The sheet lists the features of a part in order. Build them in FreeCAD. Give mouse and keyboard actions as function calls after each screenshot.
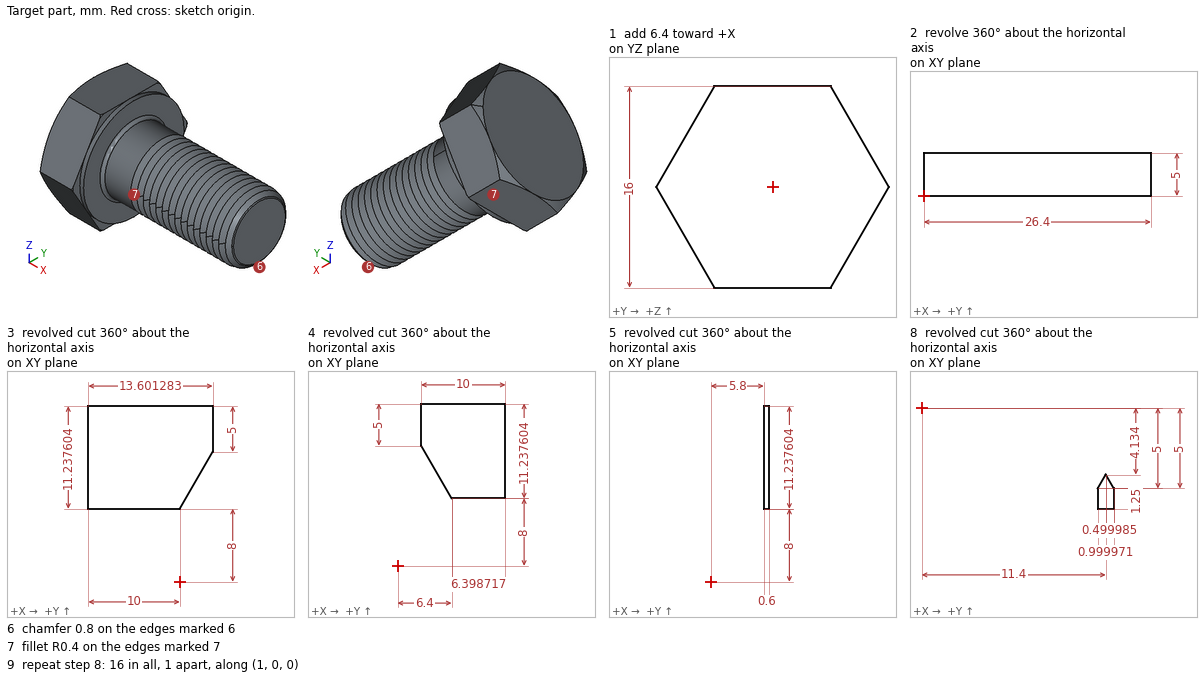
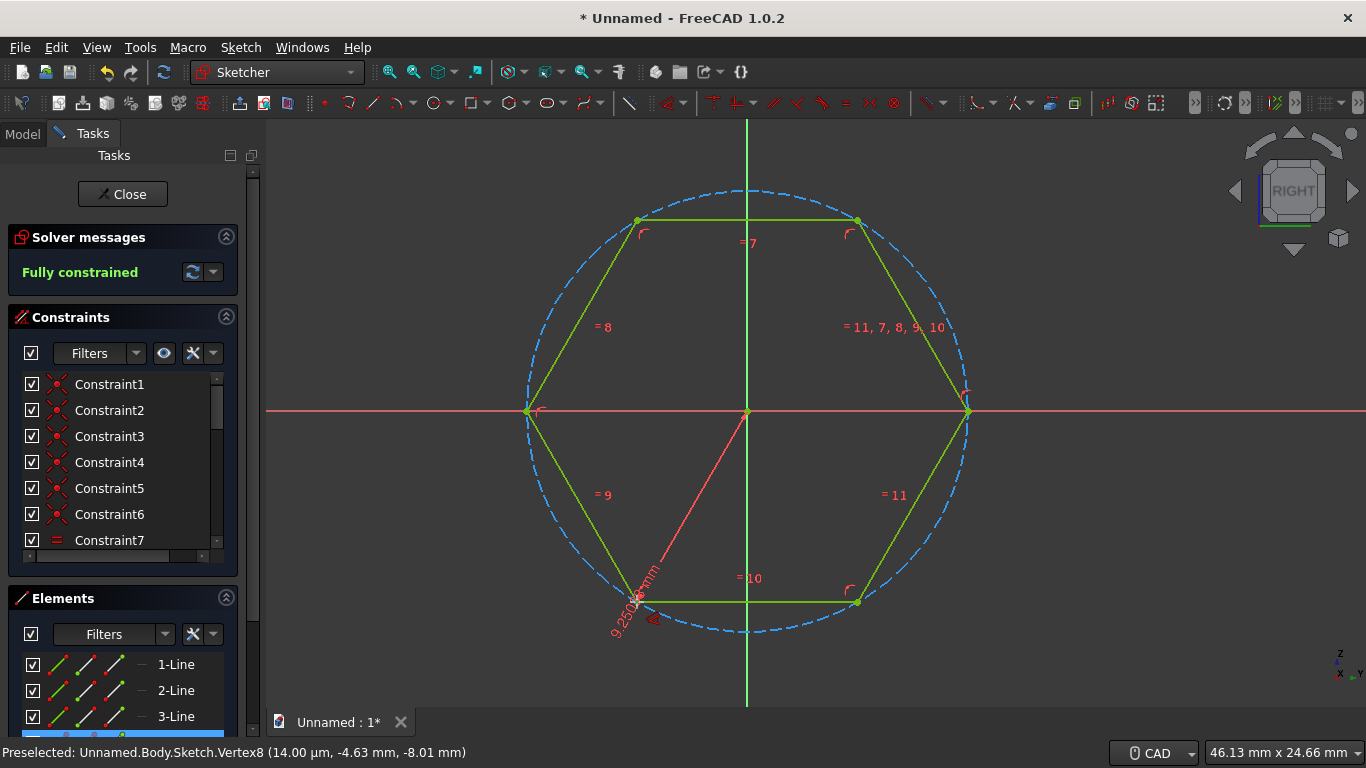
click(858, 220)
click(892, 324)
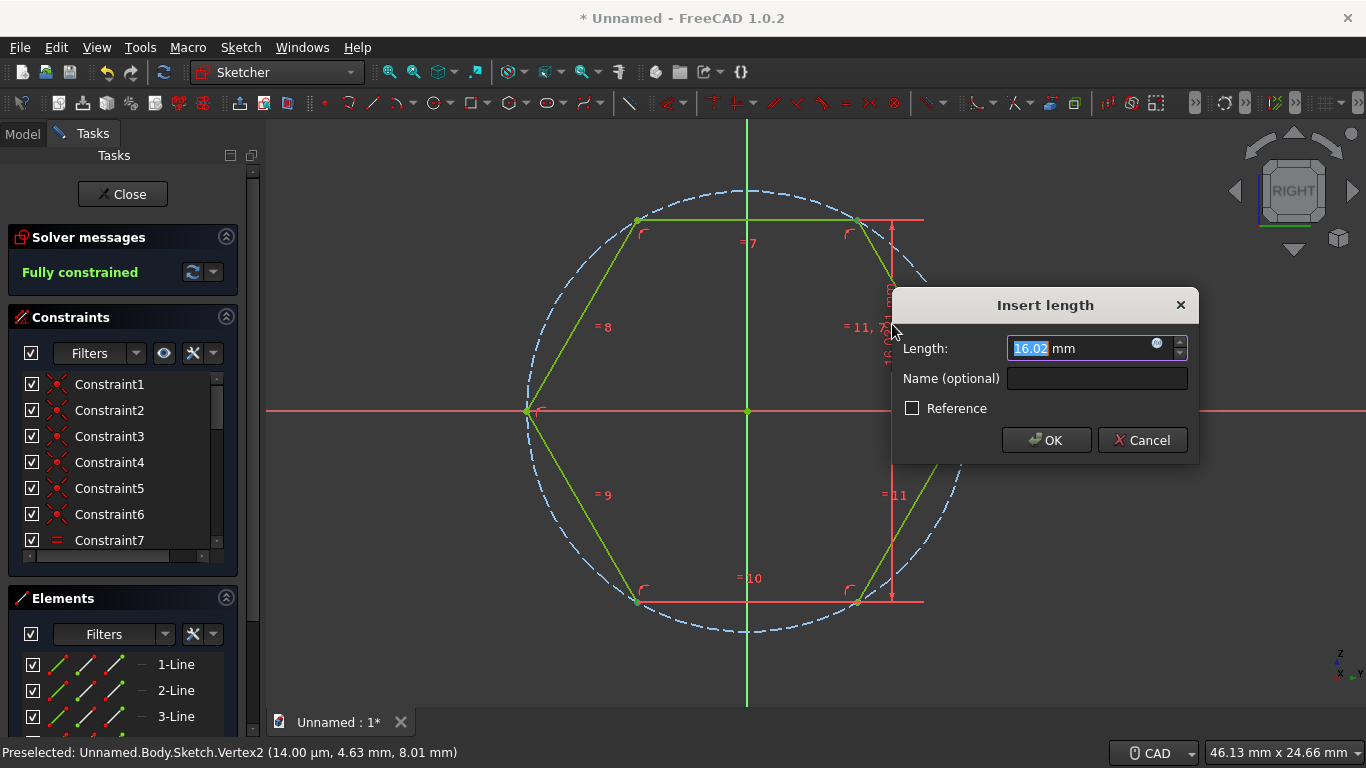
text(16)
key(Return)
key(Escape)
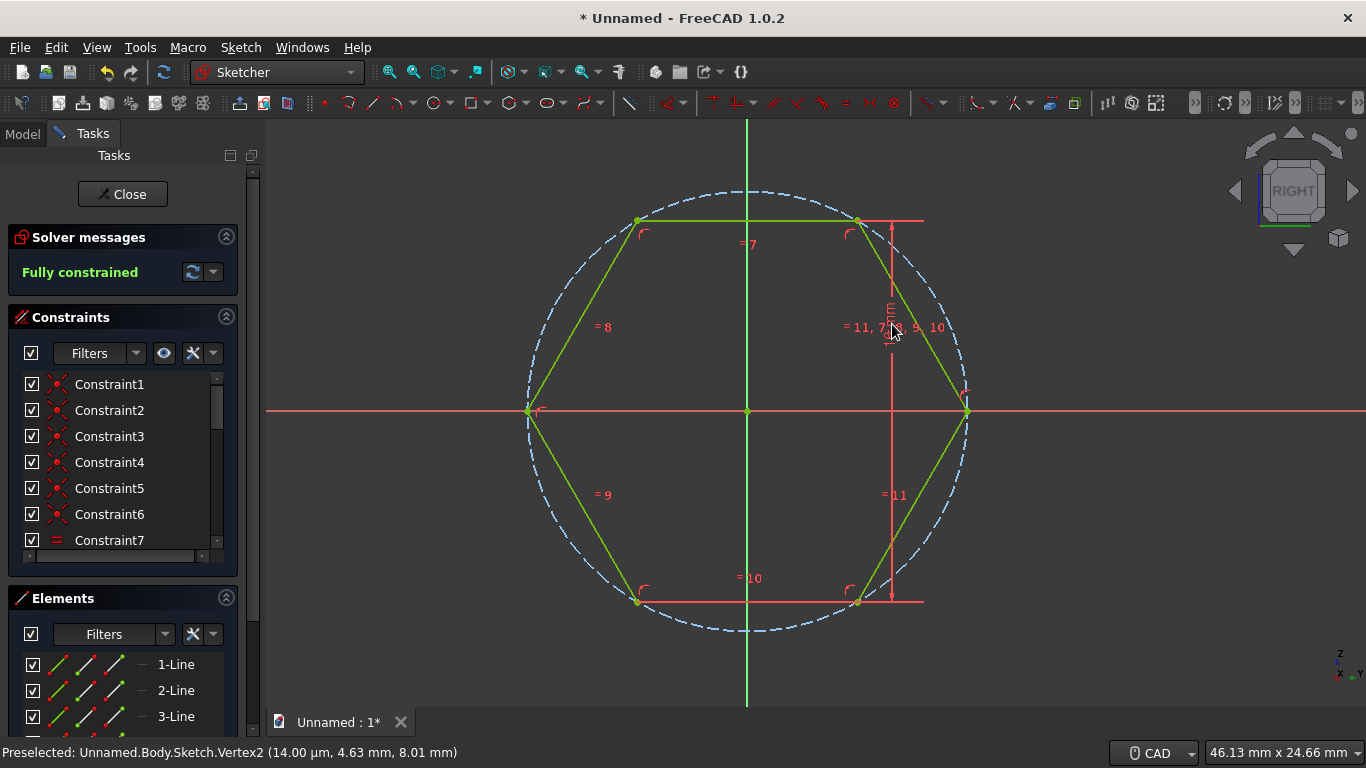
click(123, 194)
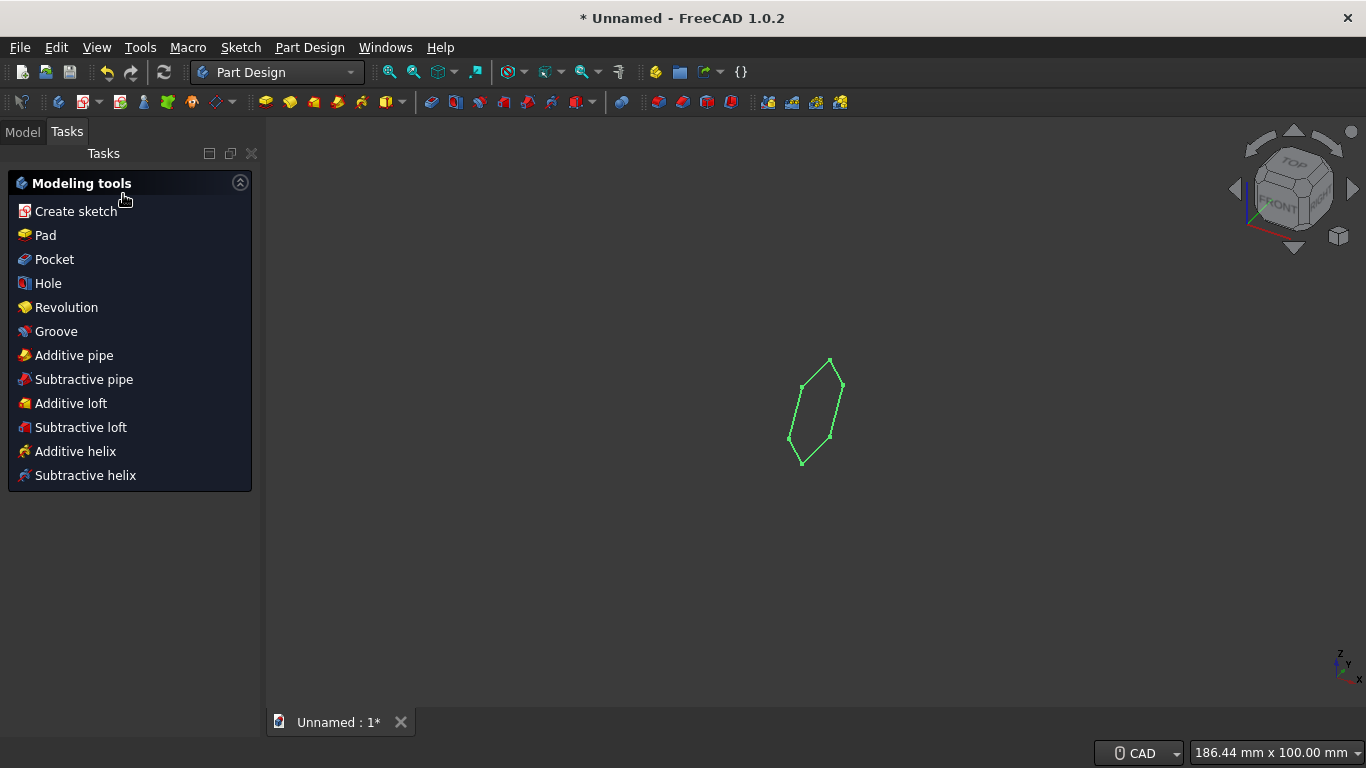
click(266, 102)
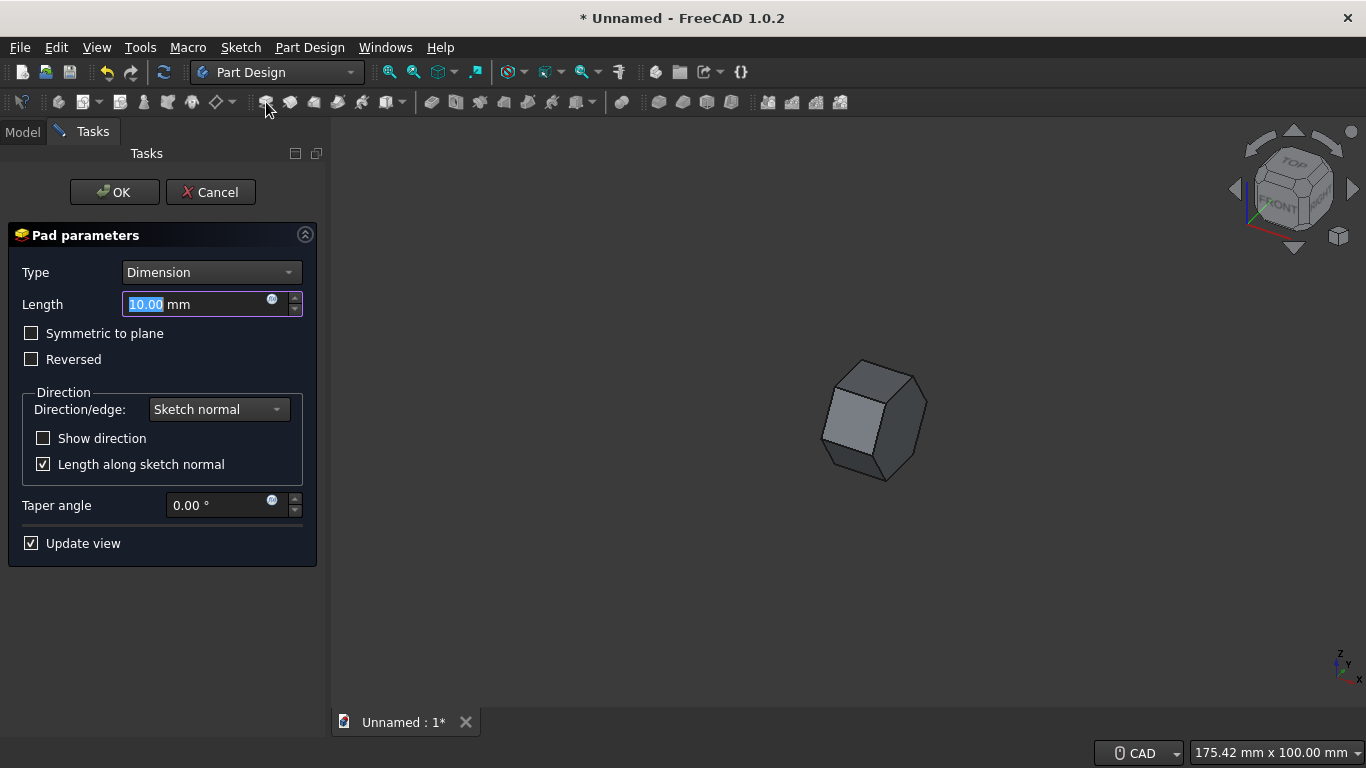
text(6.4)
key(Tab)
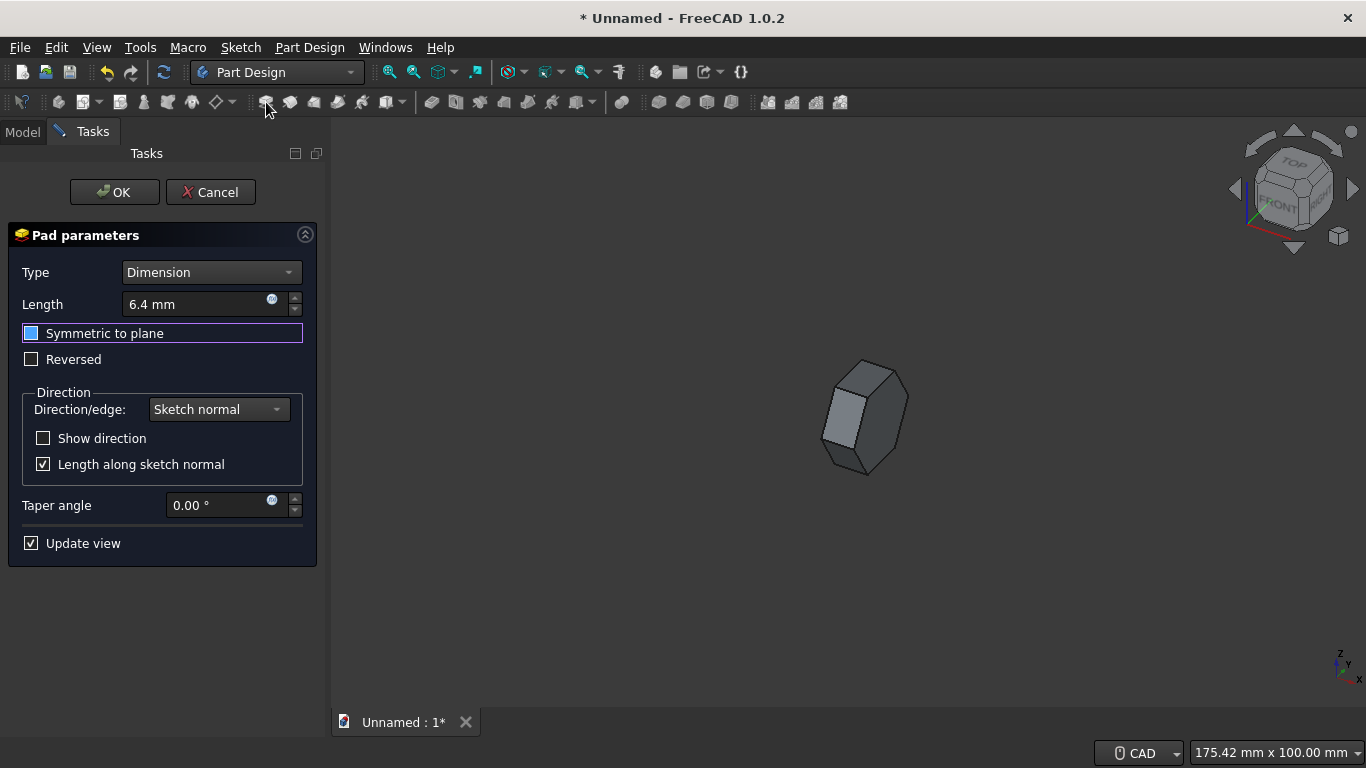
click(115, 192)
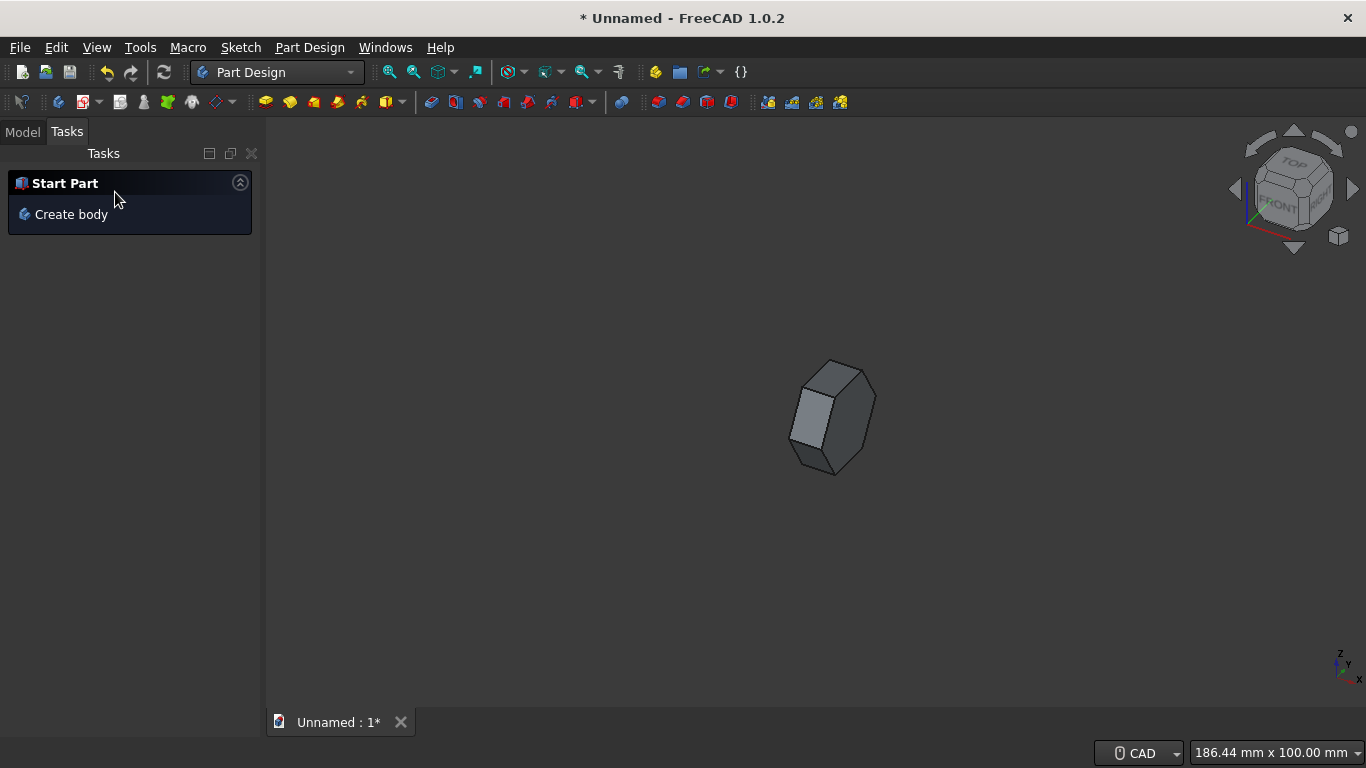
click(390, 72)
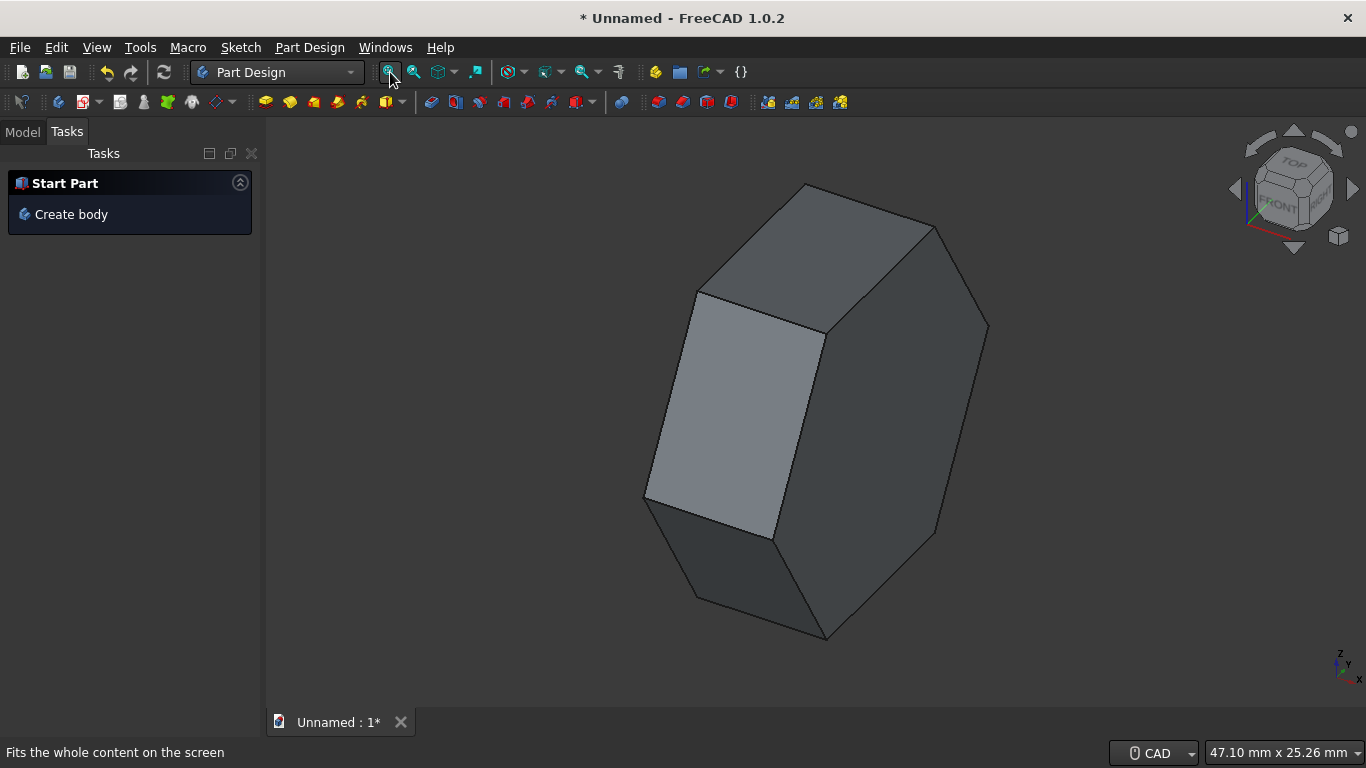
click(84, 102)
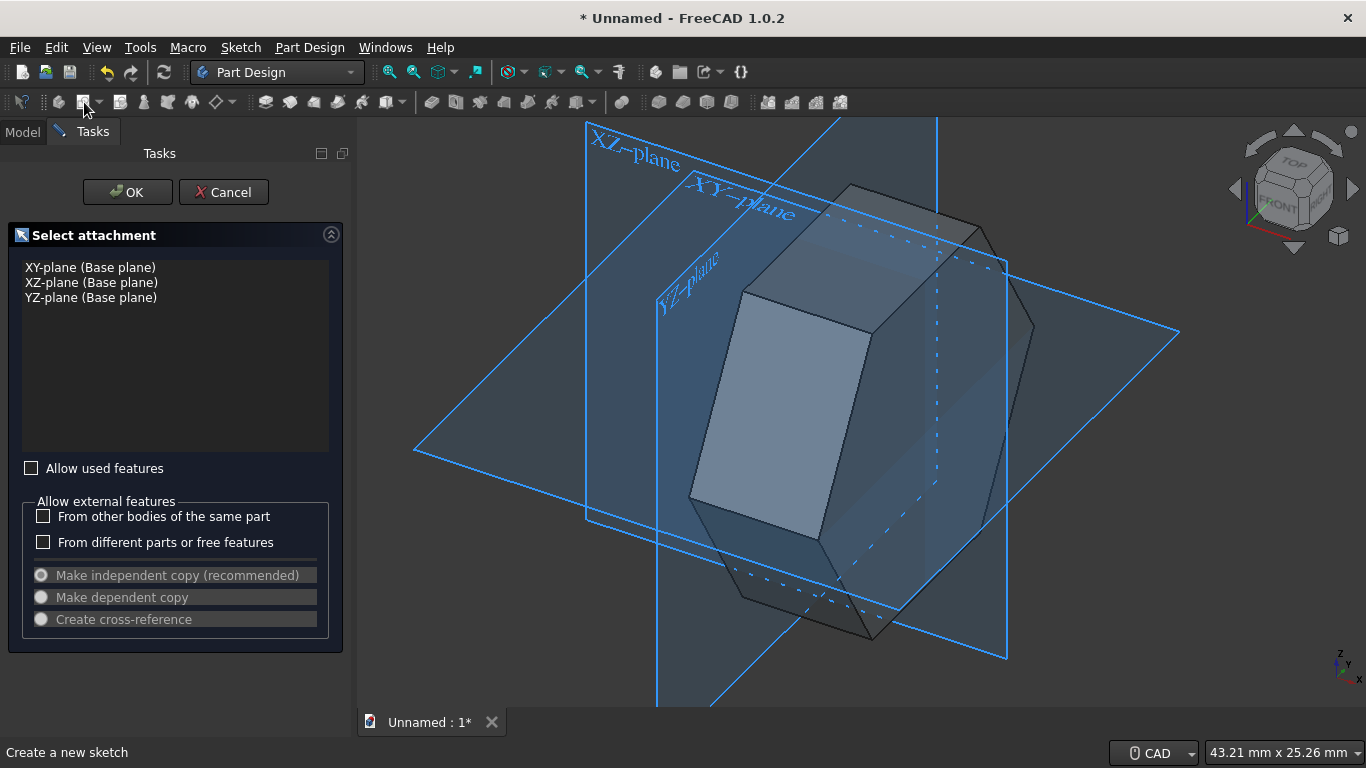
click(82, 268)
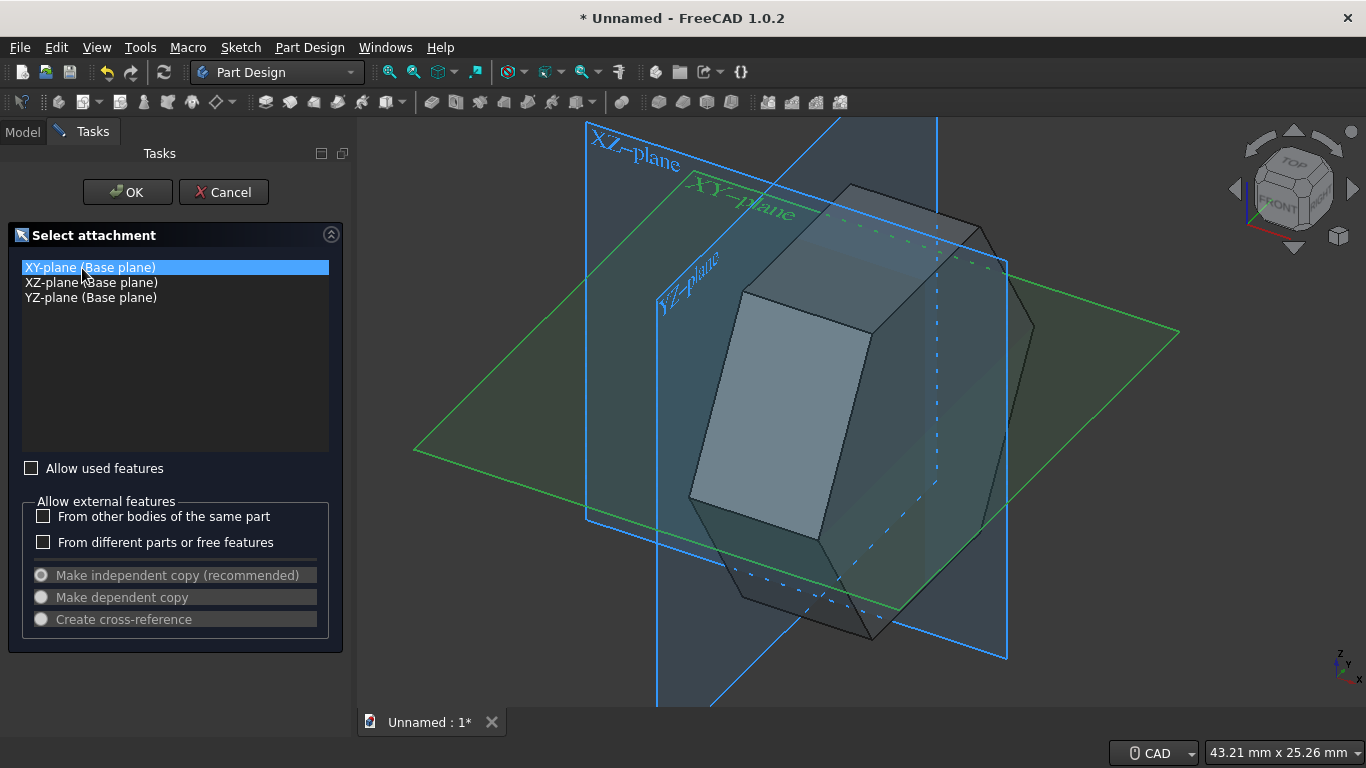
click(128, 192)